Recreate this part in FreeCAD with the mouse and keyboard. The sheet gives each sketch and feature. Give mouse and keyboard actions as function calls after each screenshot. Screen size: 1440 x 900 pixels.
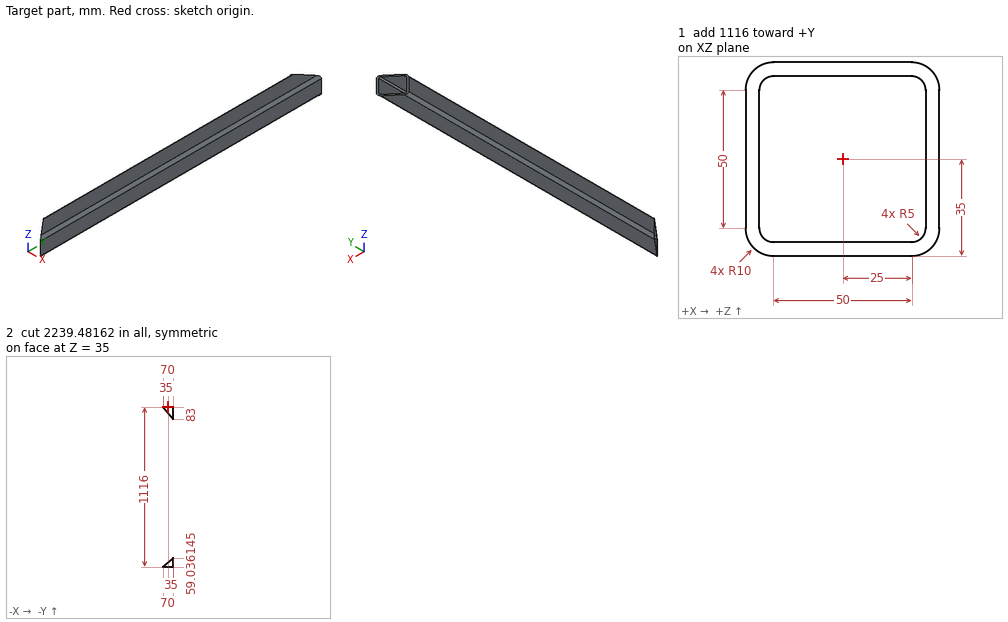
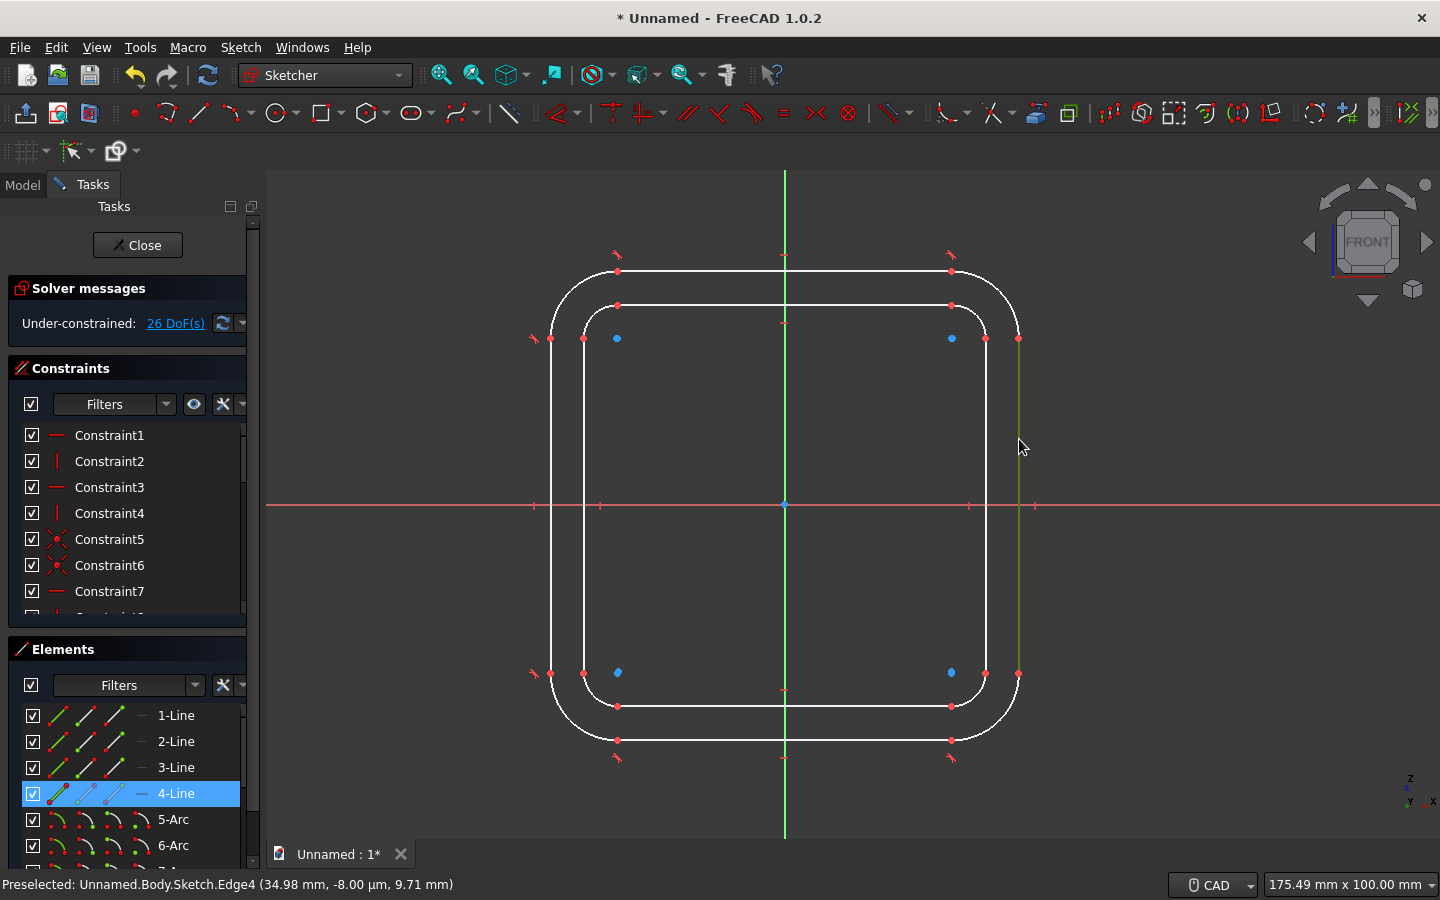
click(1012, 308)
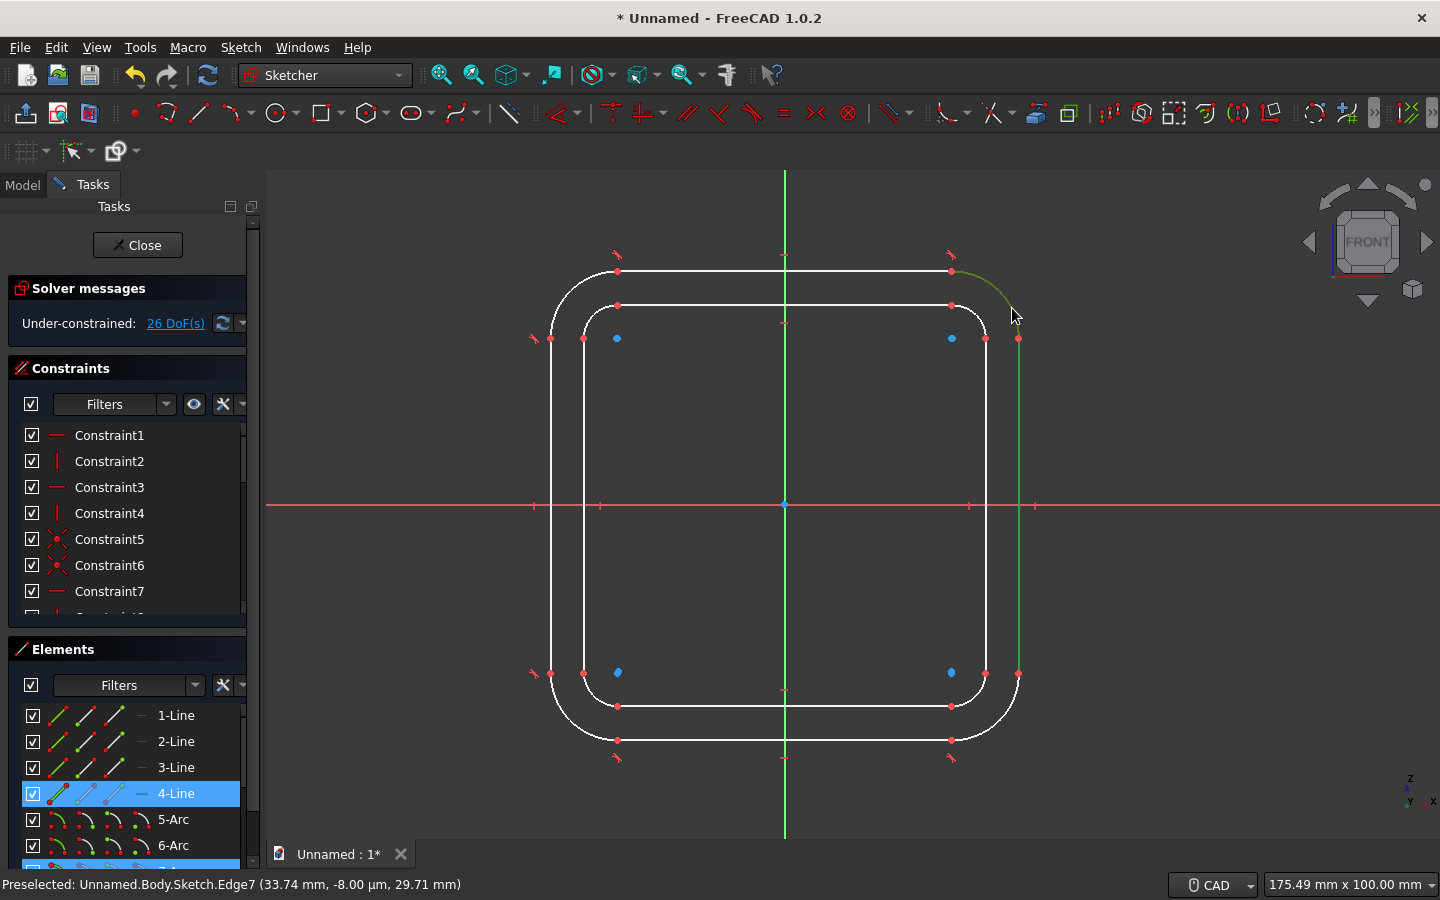
click(752, 114)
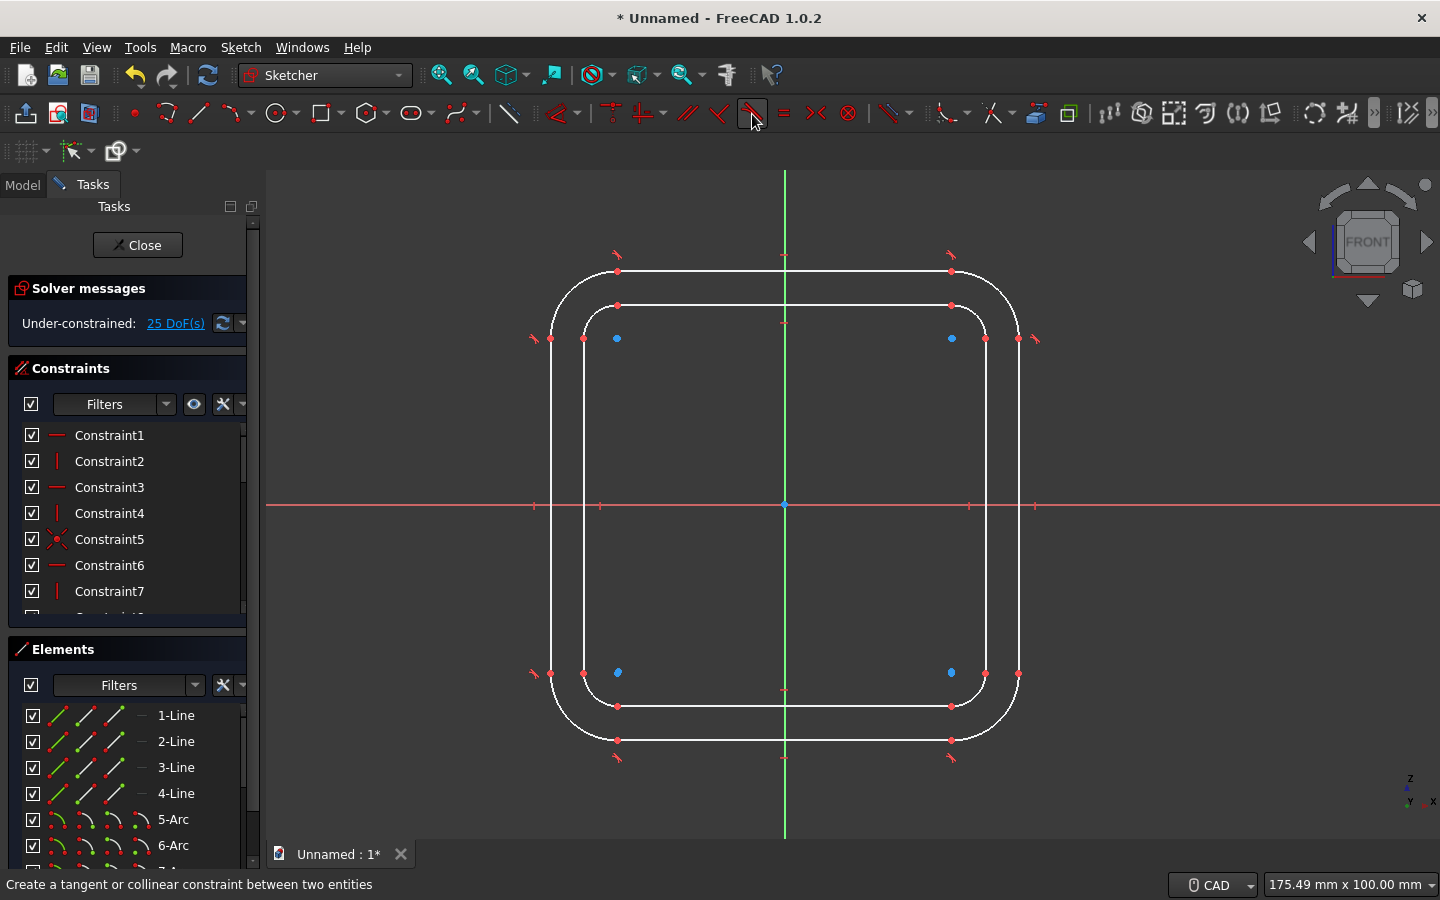
click(1019, 439)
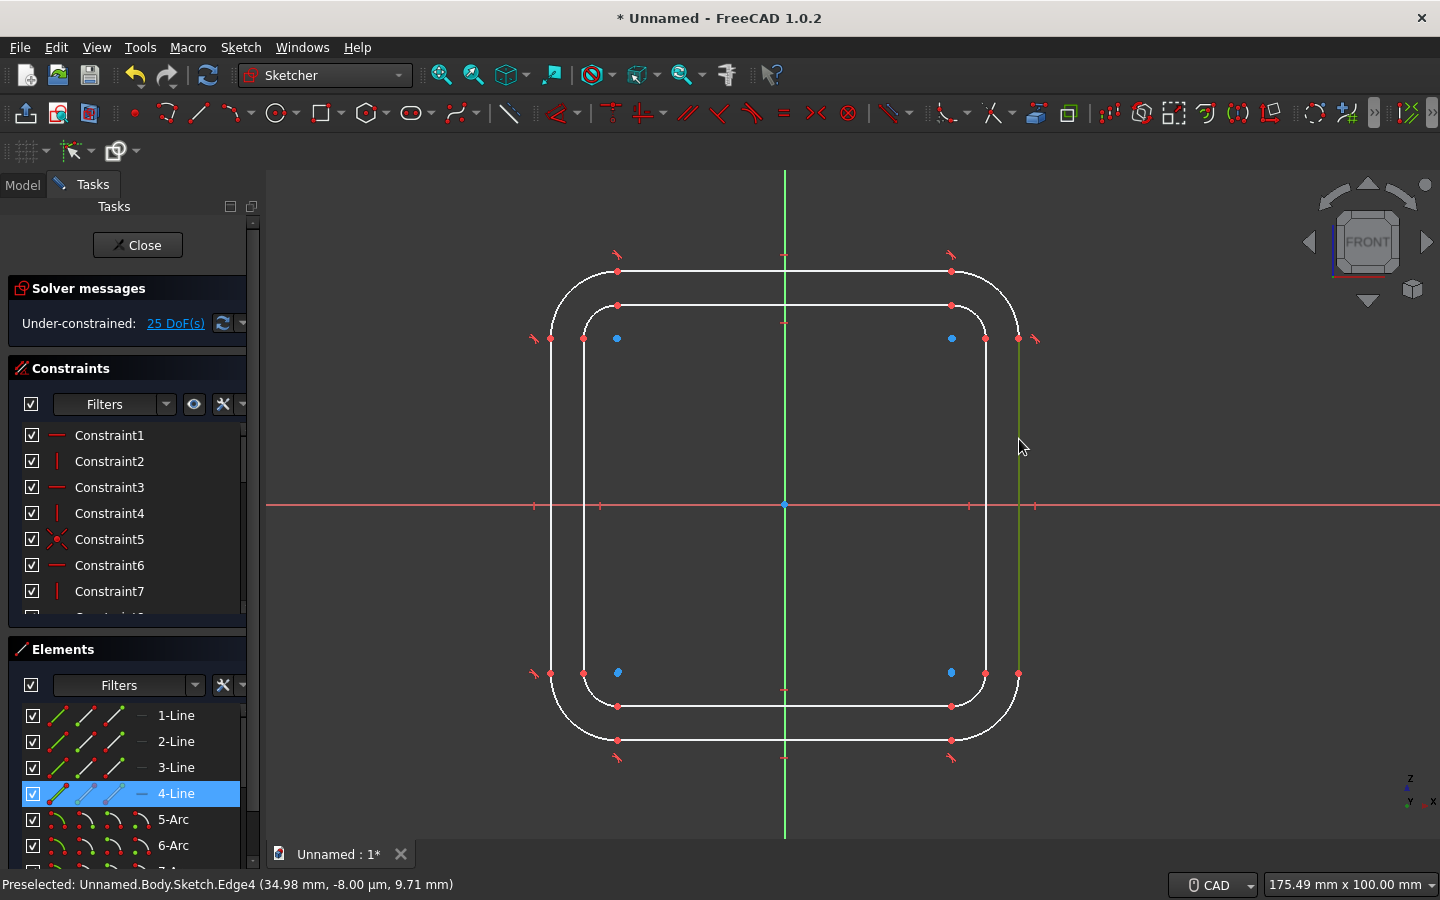
click(982, 733)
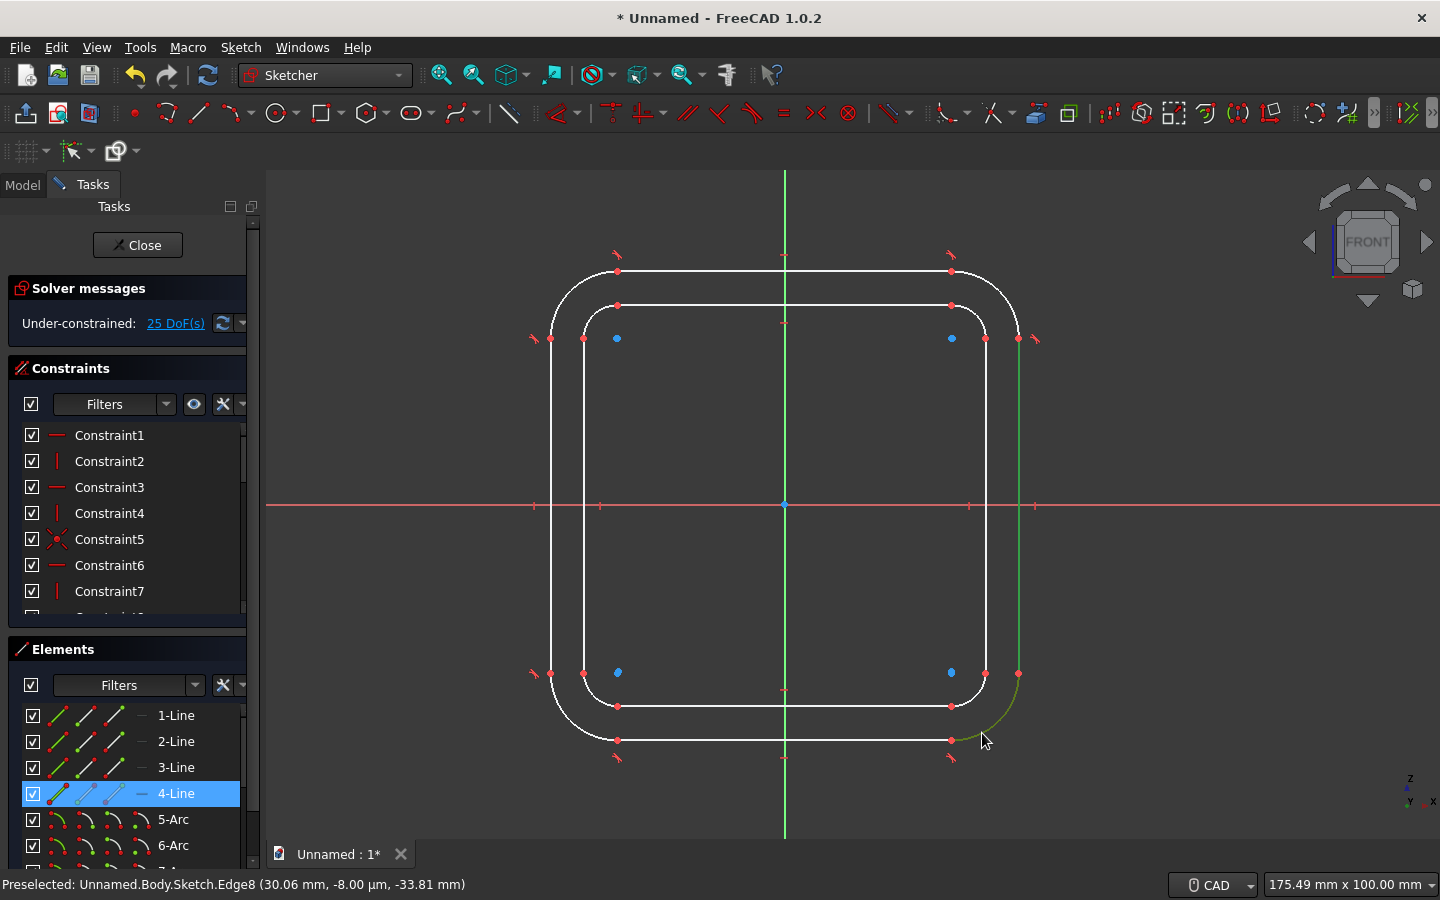
click(752, 114)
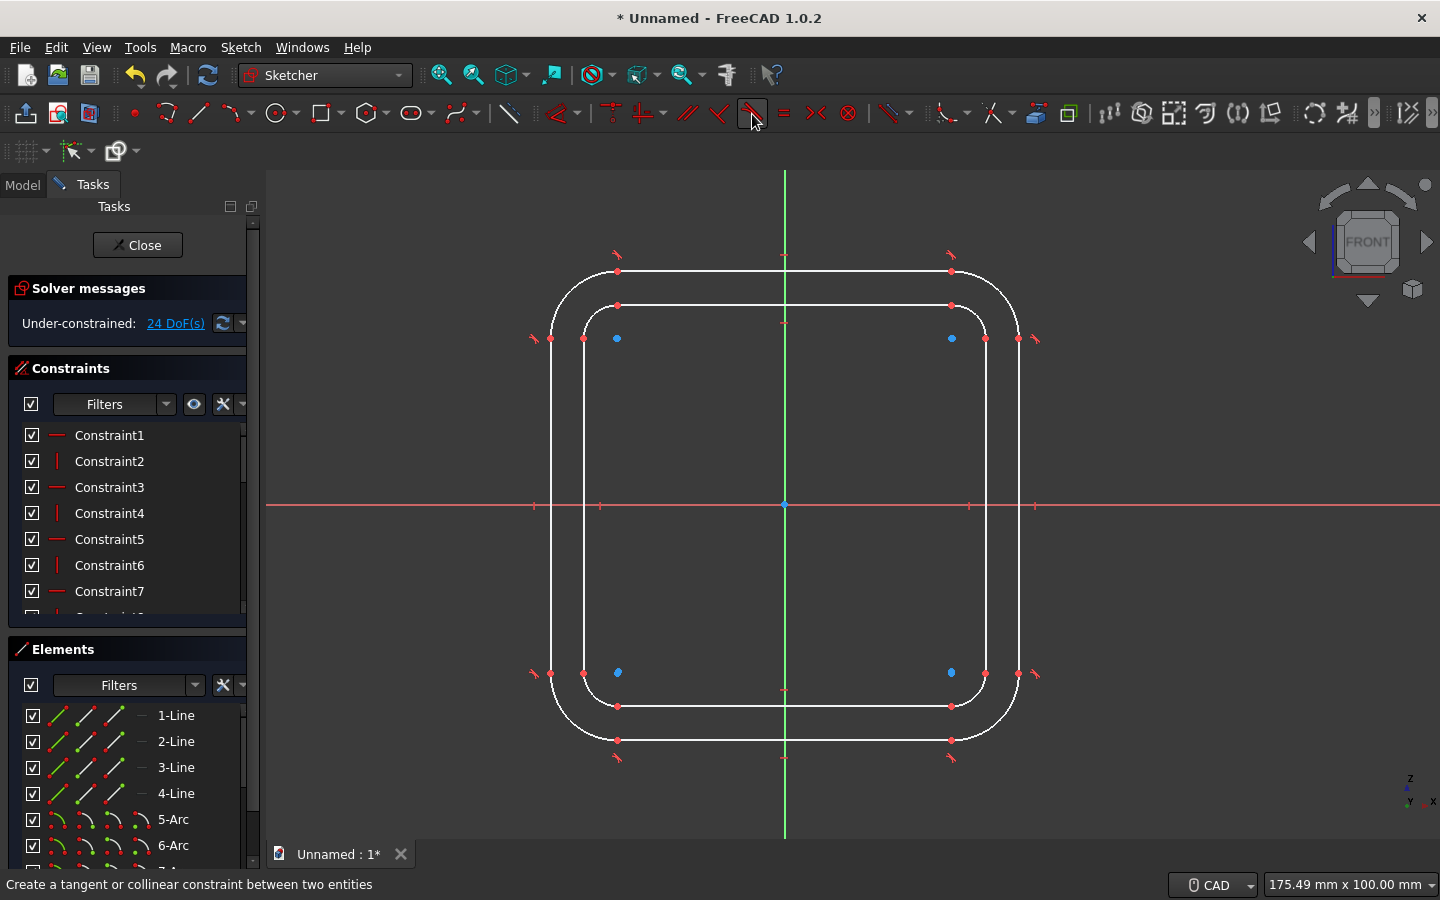
click(718, 706)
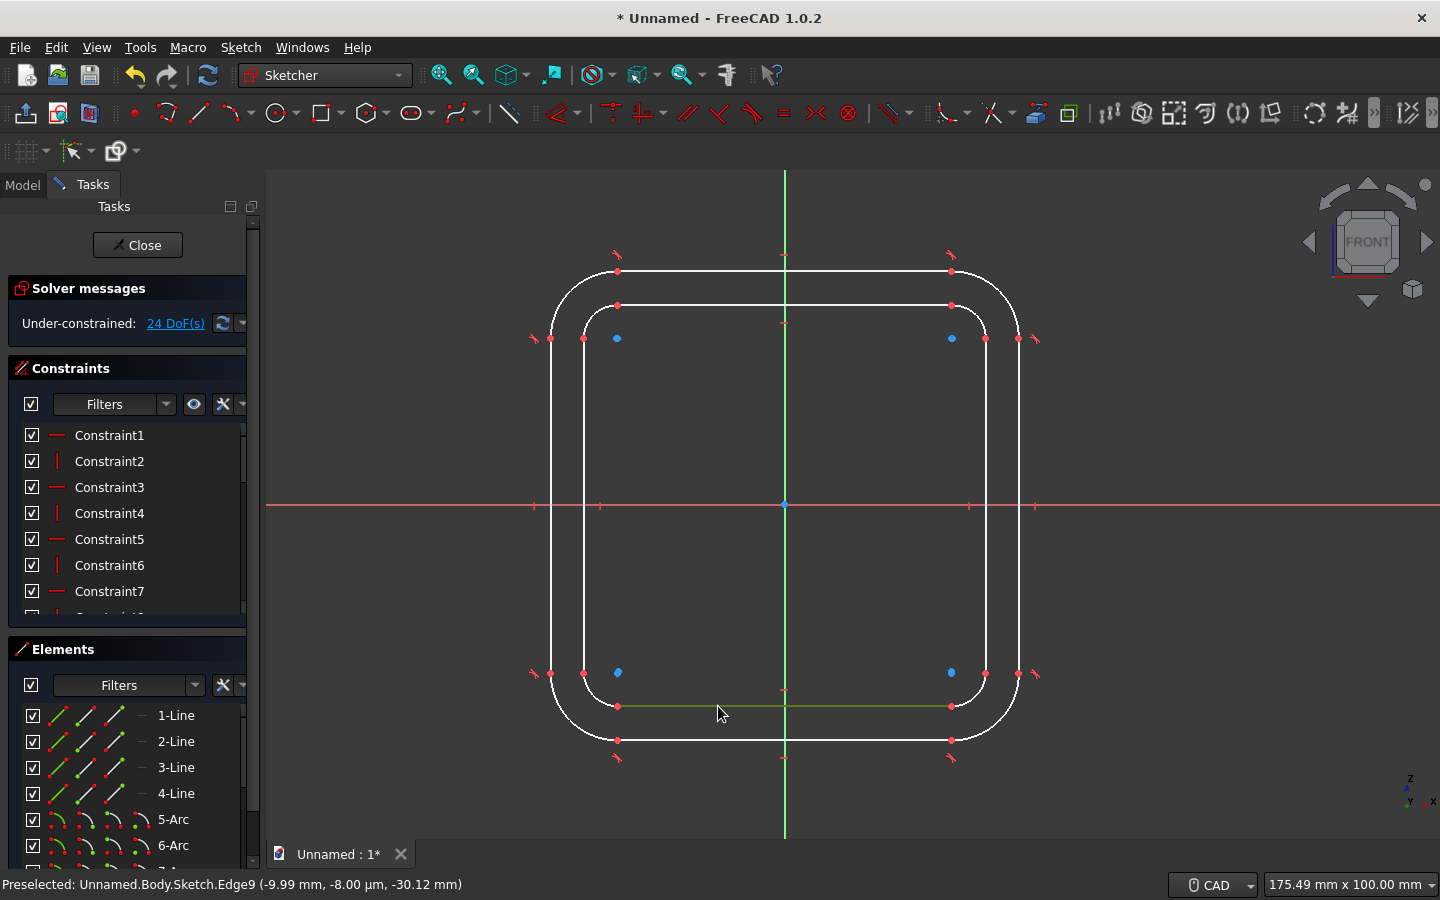
click(967, 703)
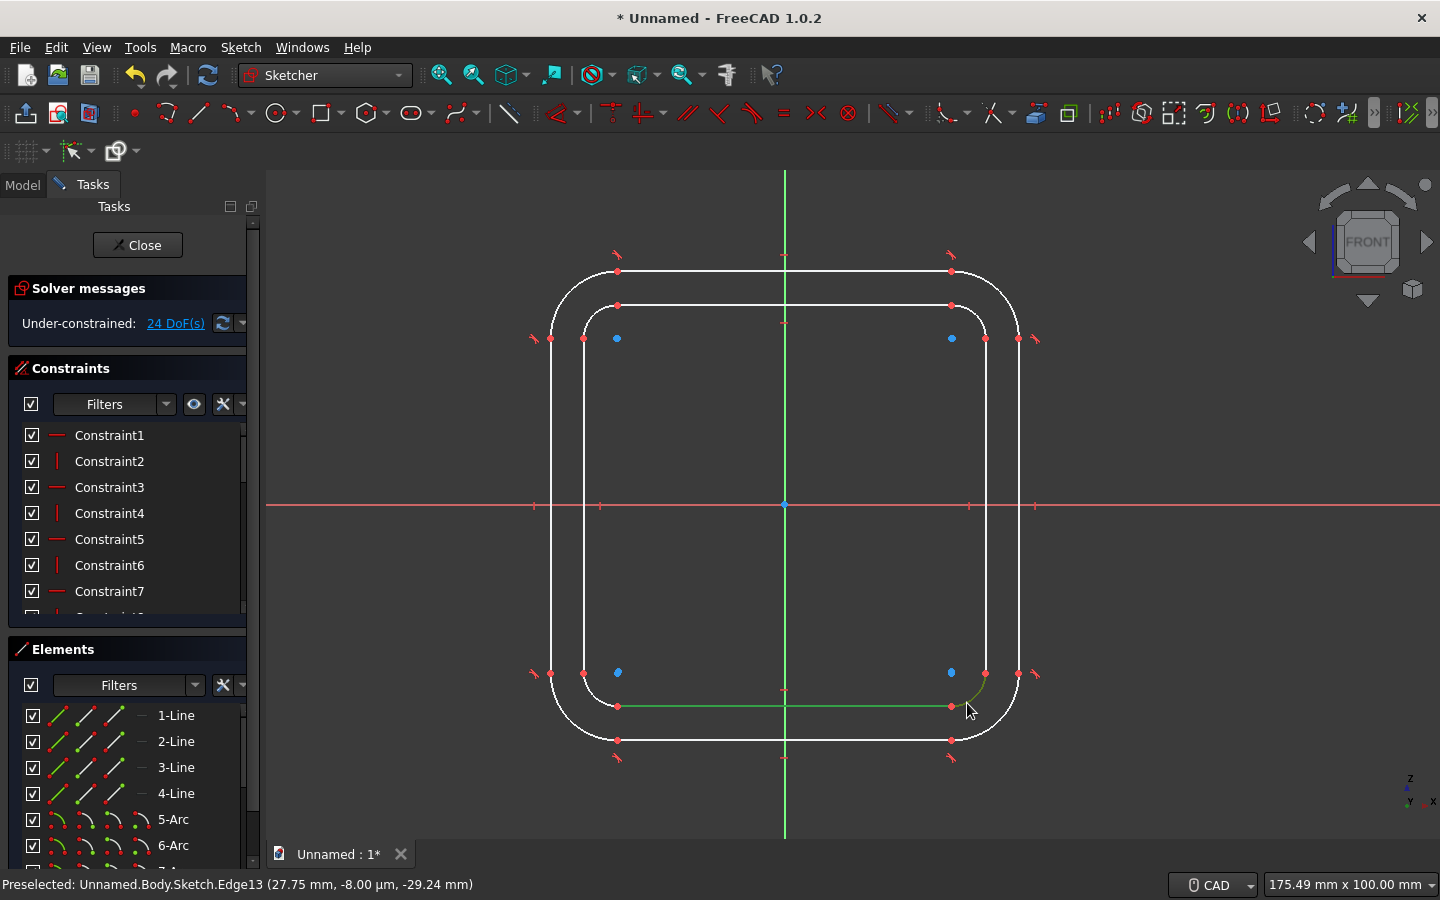
key(t)